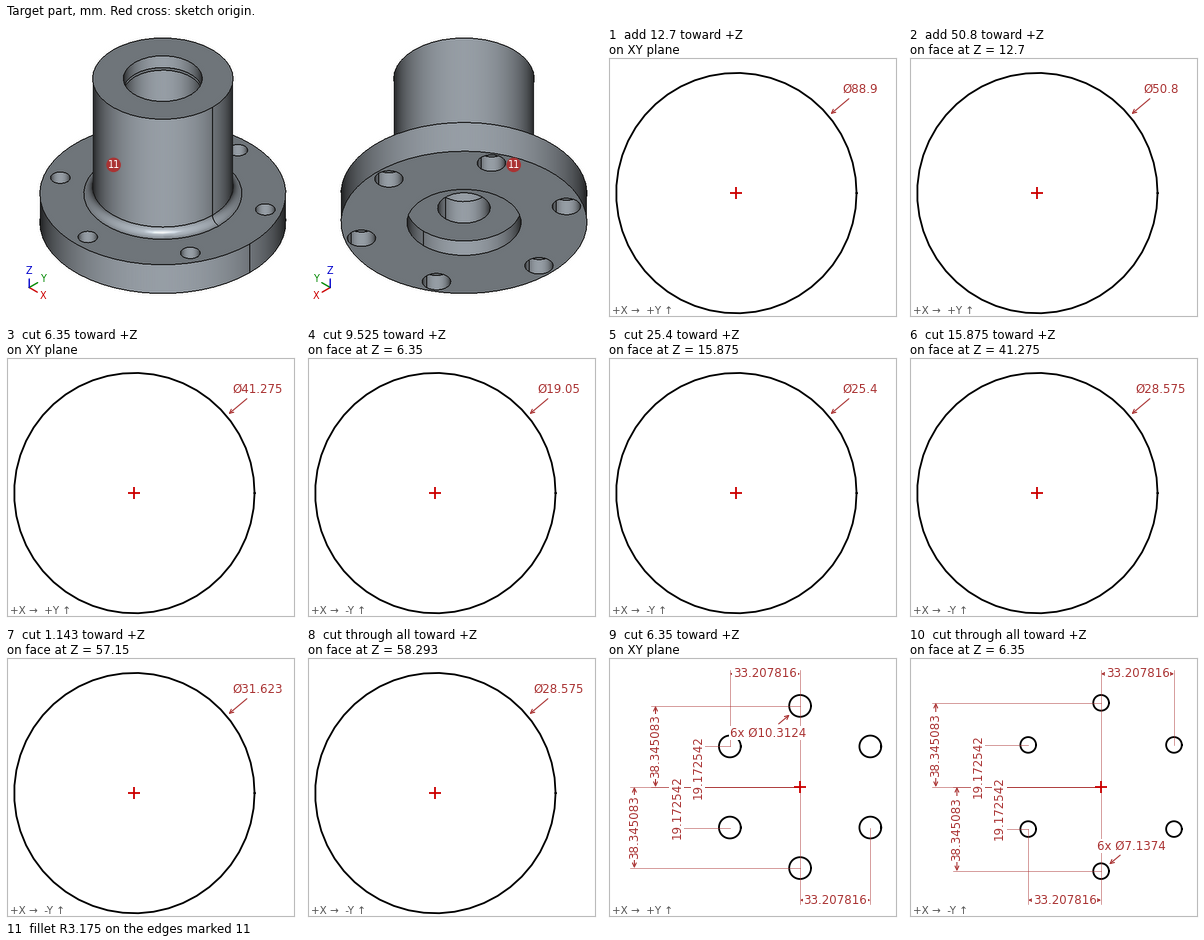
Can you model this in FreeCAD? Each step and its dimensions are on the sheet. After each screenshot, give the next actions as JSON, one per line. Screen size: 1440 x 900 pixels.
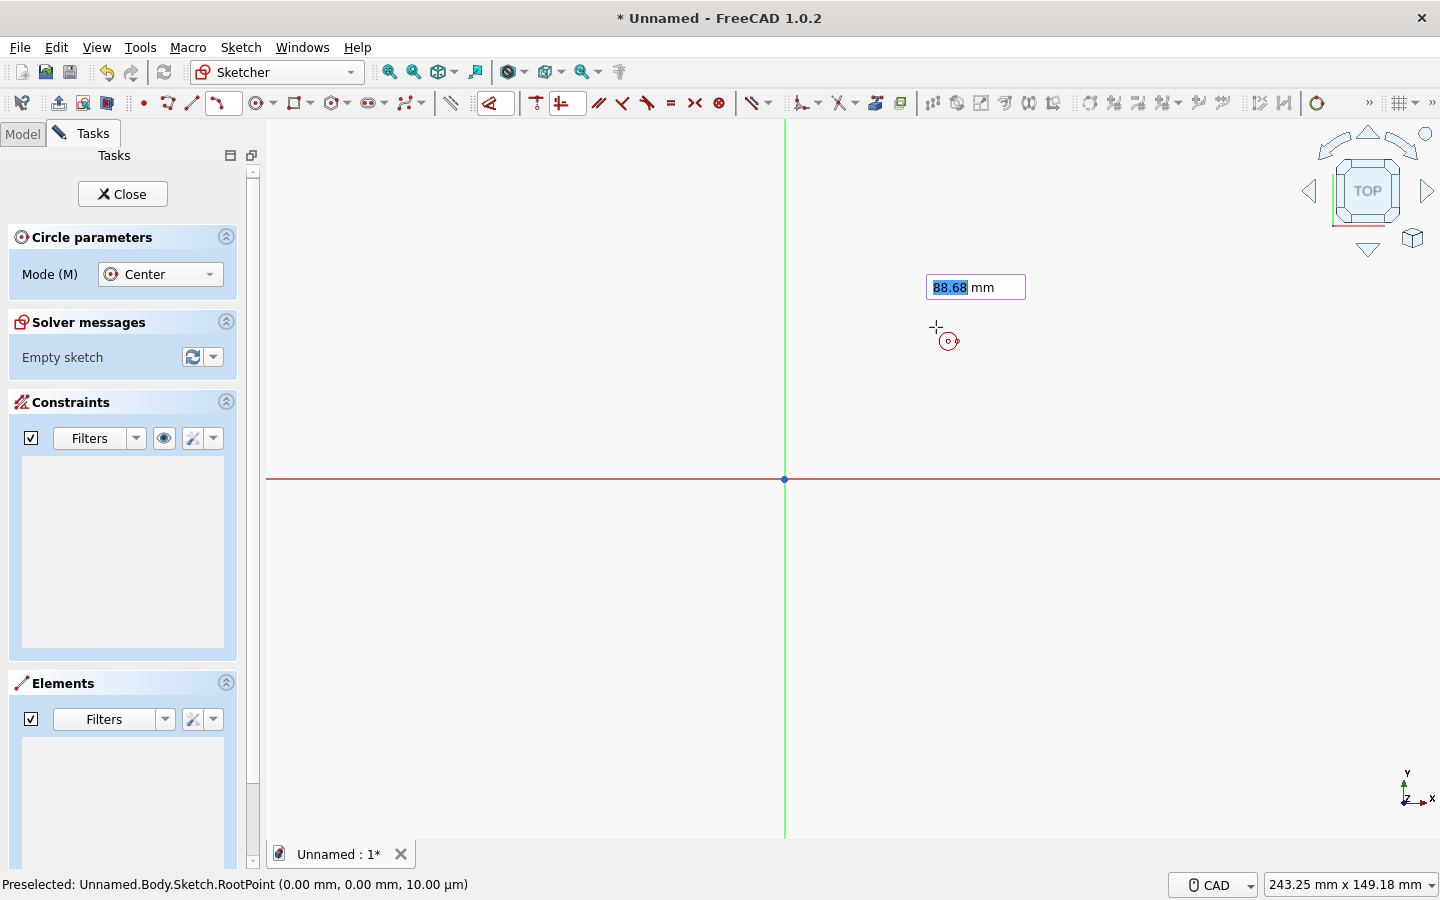
{"action": "type", "text": "88.9"}
{"action": "key", "text": "Return"}
{"action": "key", "text": "Escape"}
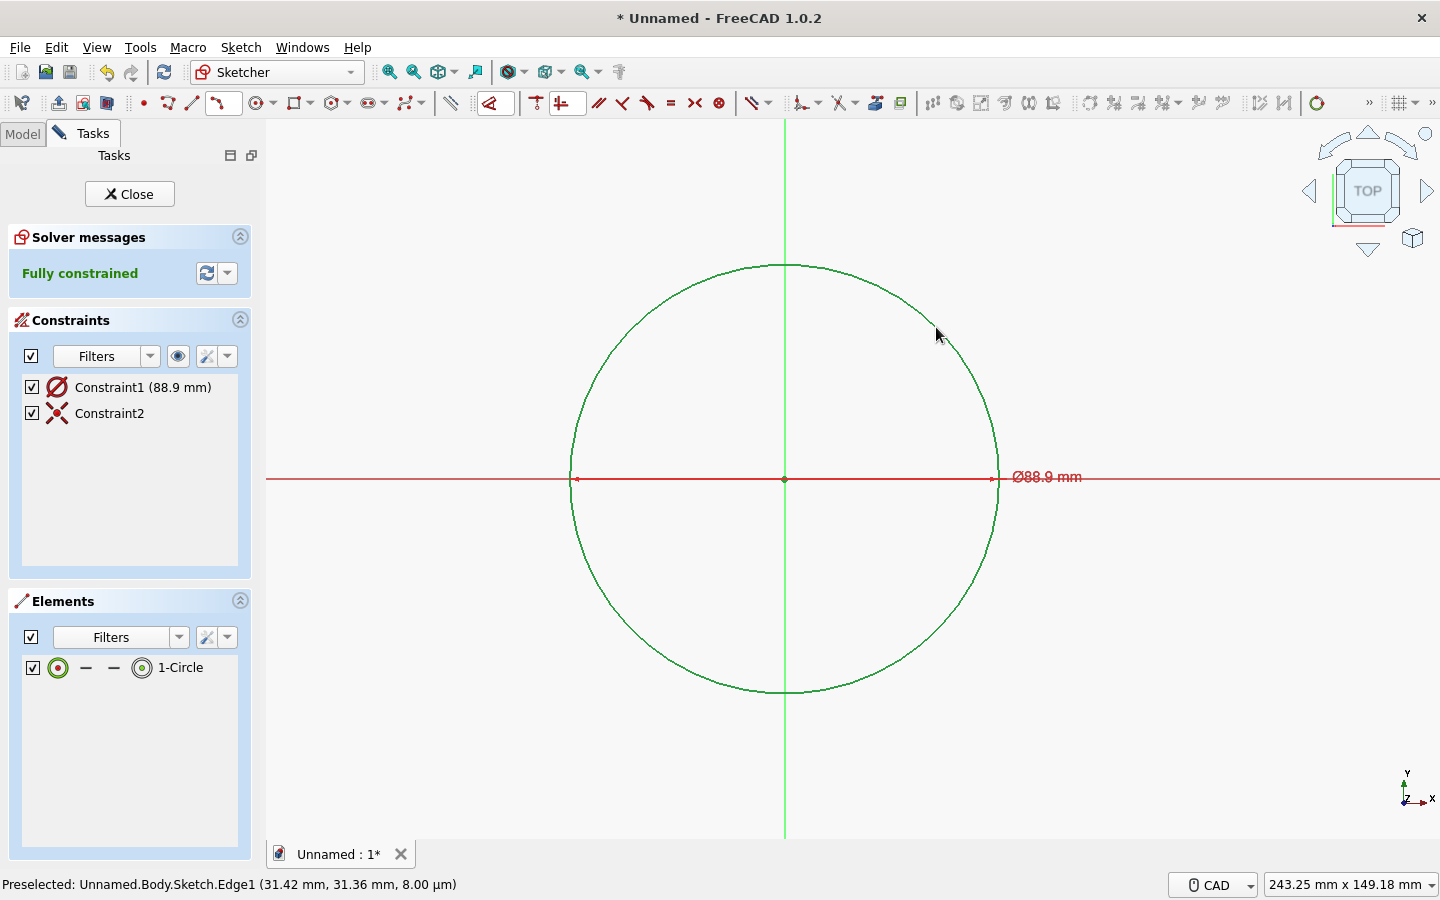
{"action": "left_click", "coordinate": [130, 194]}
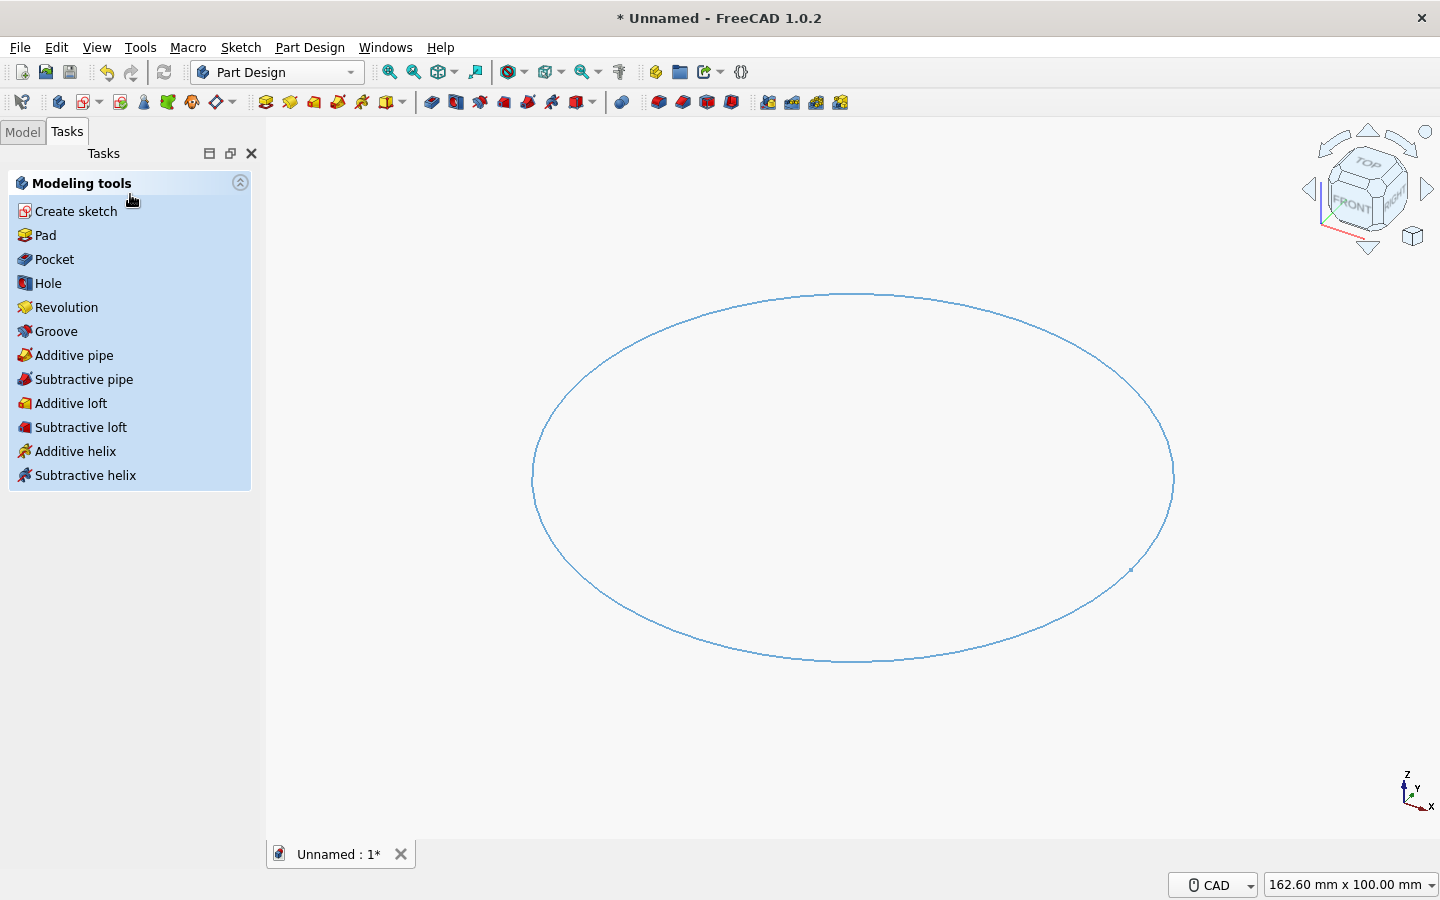
{"action": "left_click", "coordinate": [266, 102]}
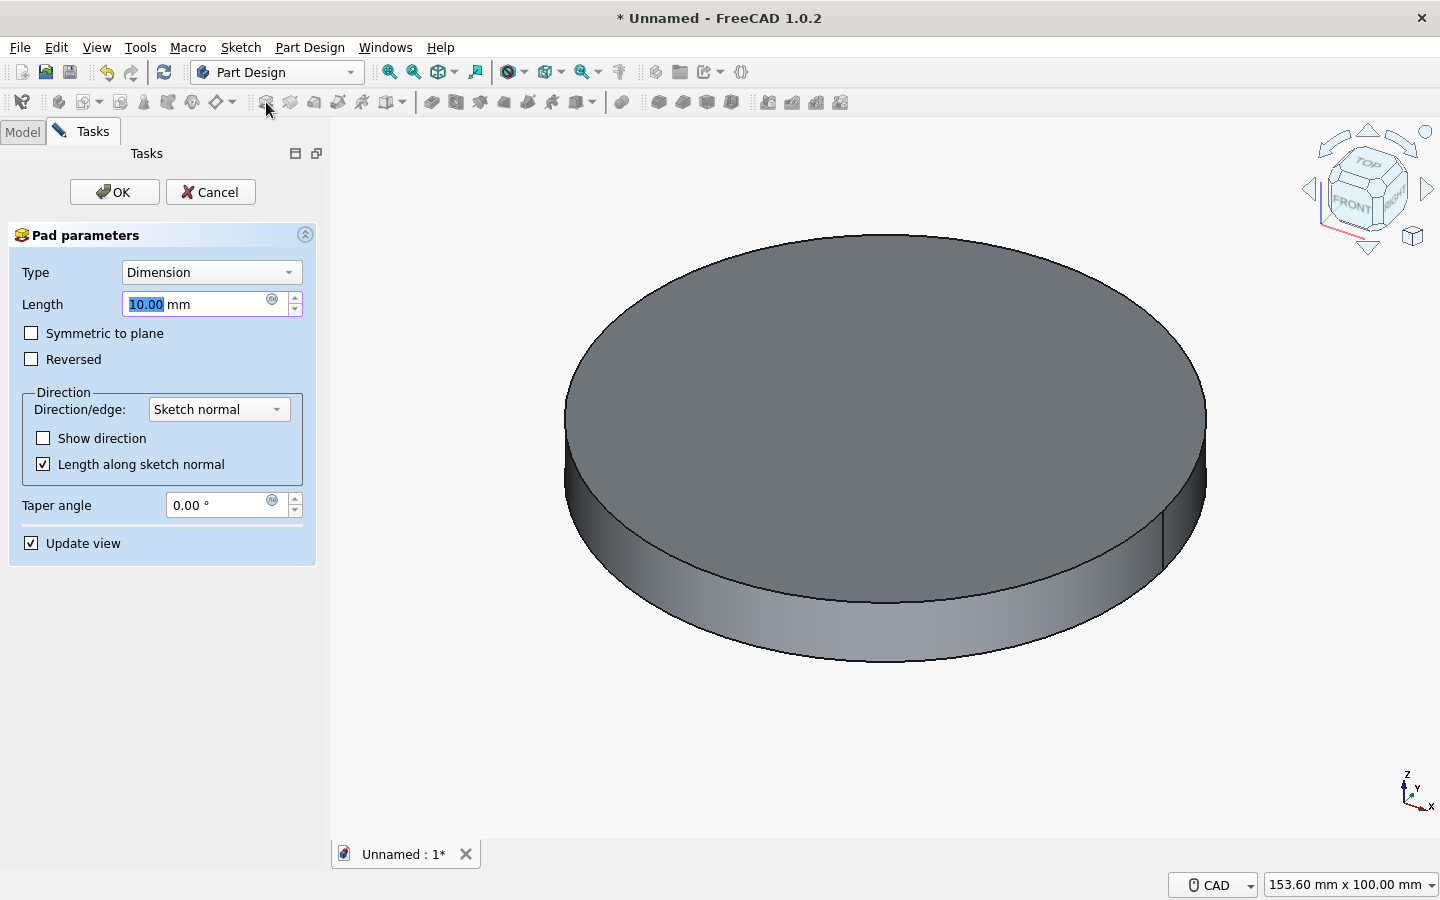
{"action": "type", "text": "12.7"}
{"action": "key", "text": "Tab"}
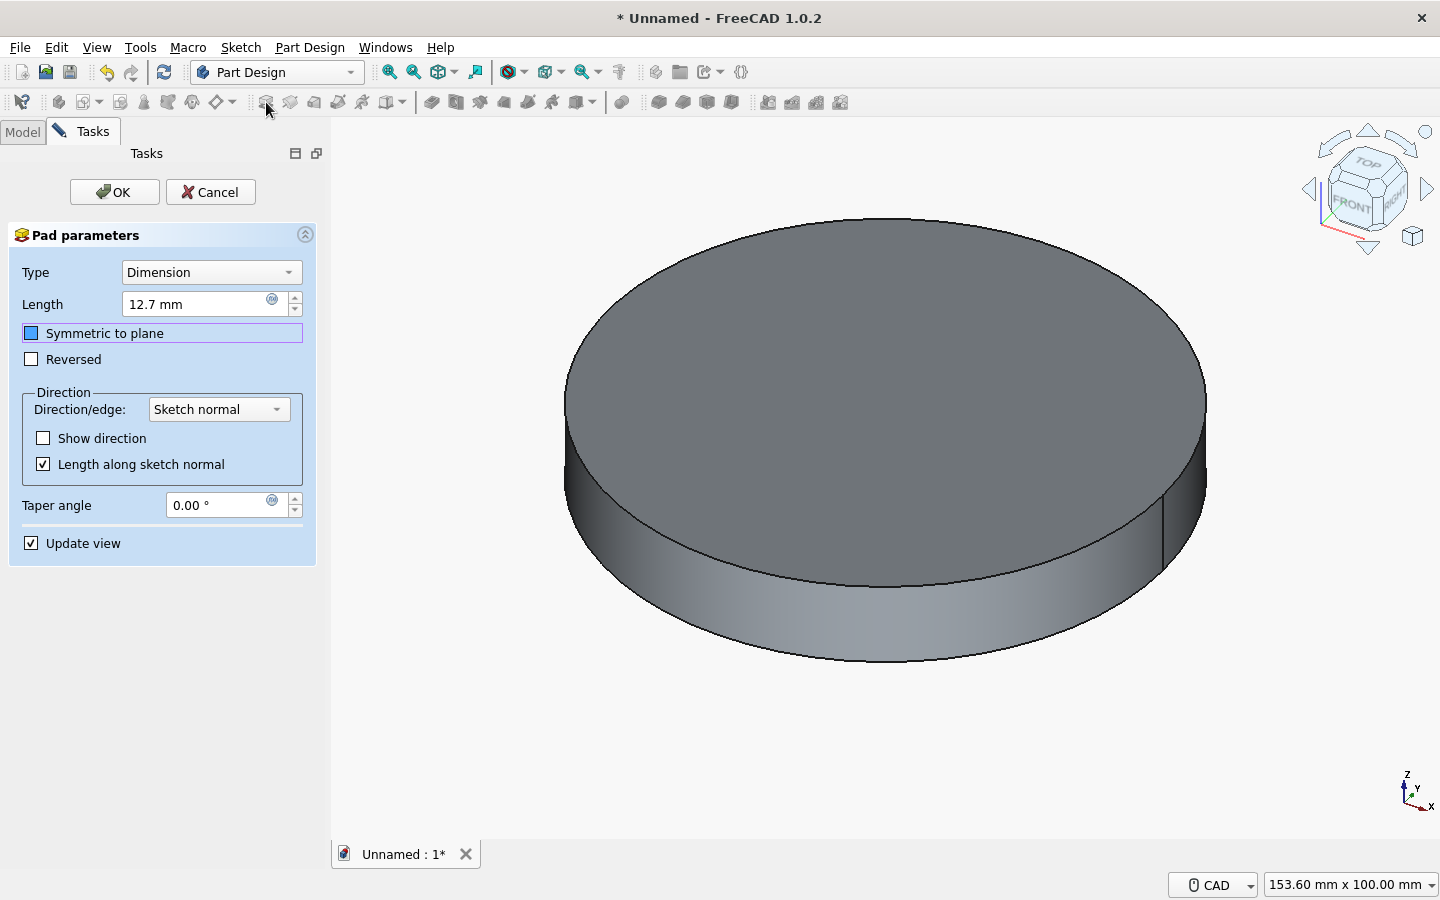
{"action": "left_click", "coordinate": [115, 192]}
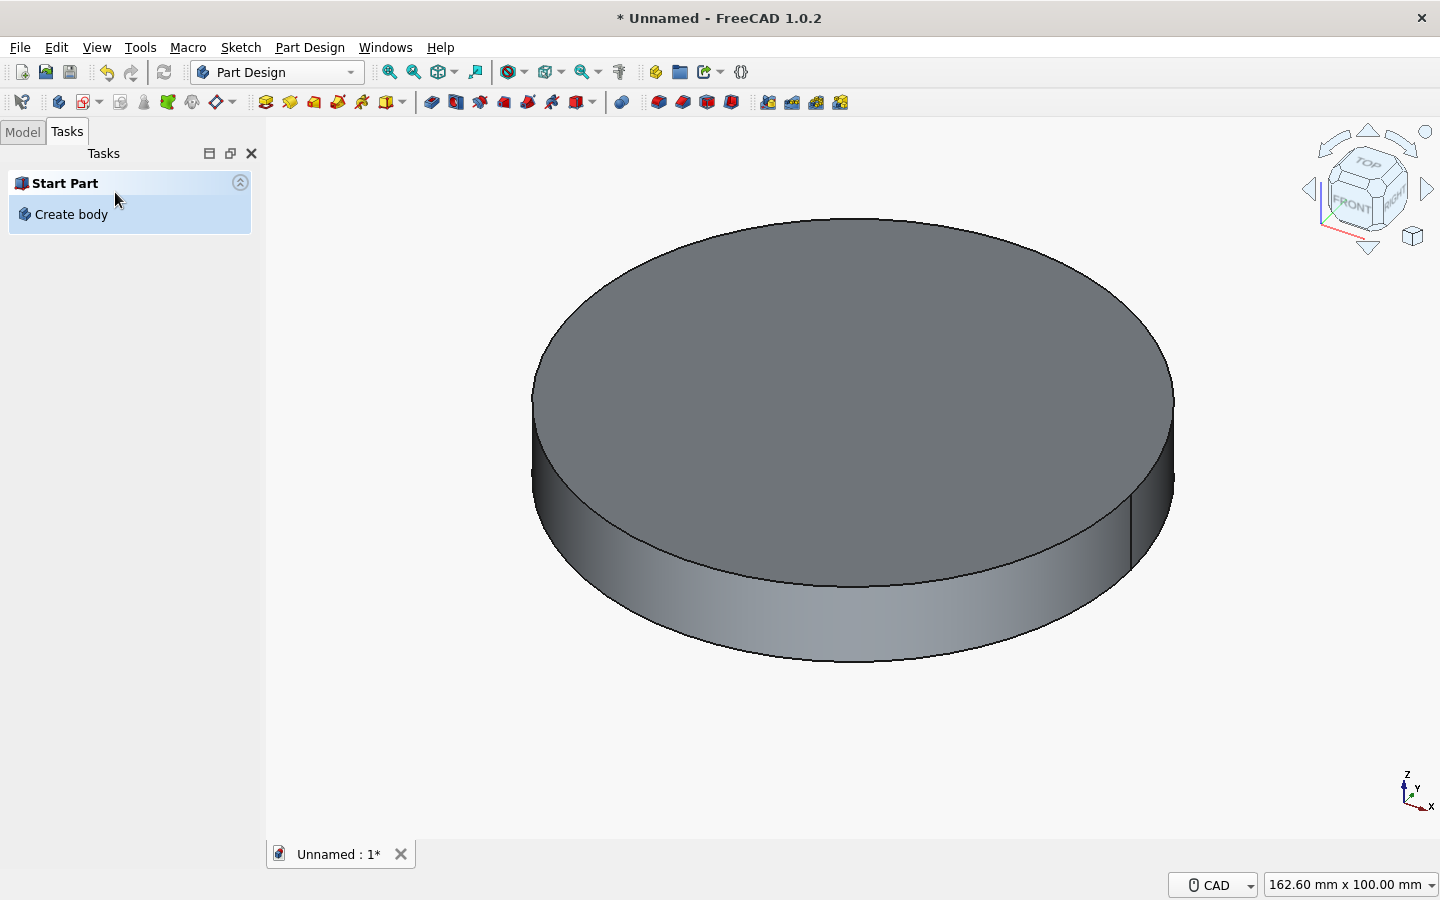
{"action": "left_click", "coordinate": [853, 402]}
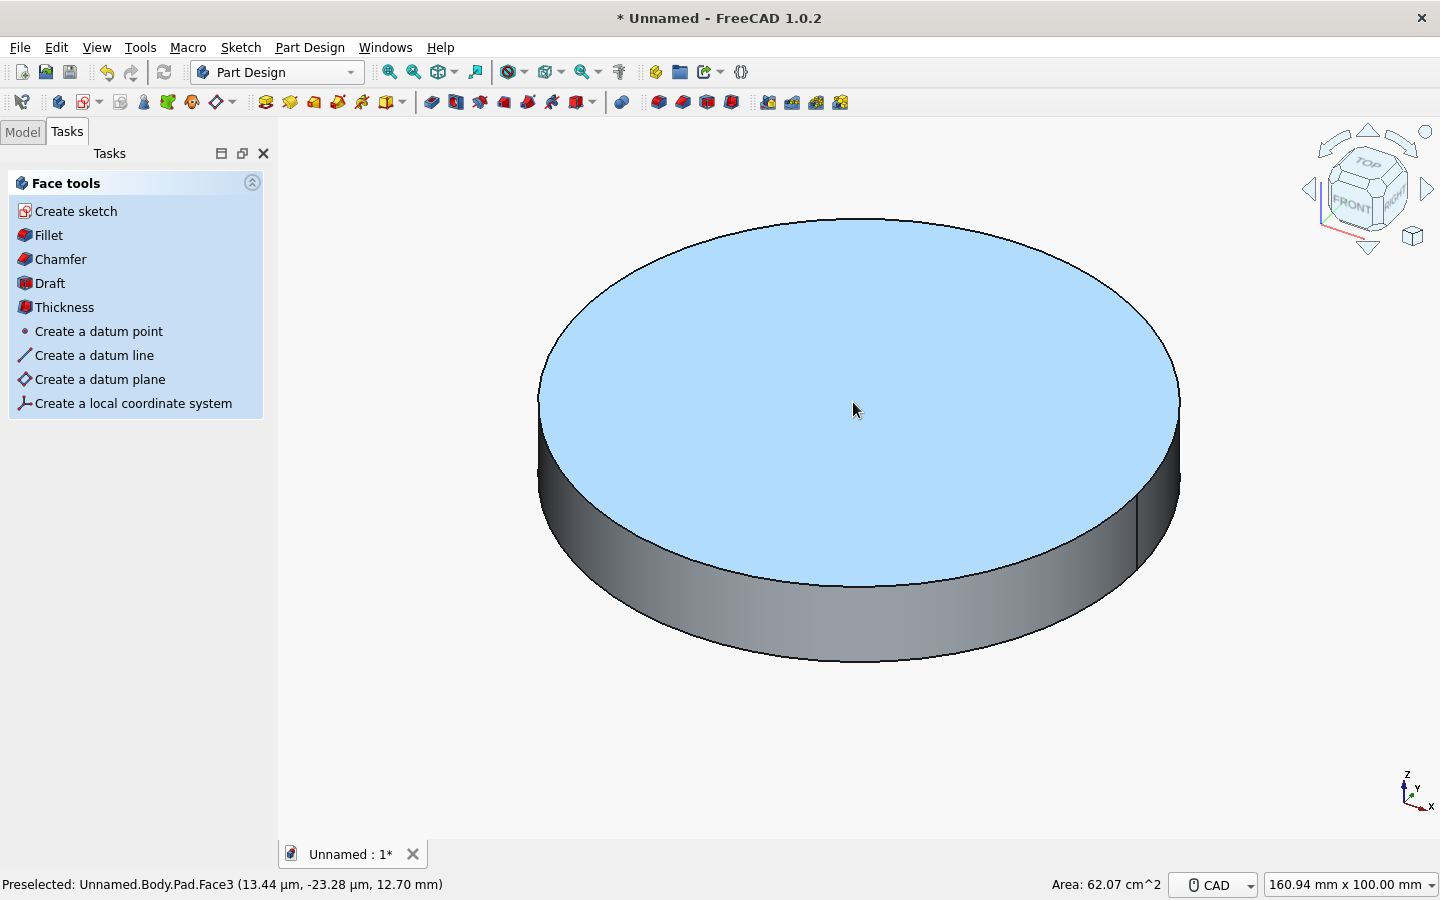
{"action": "left_click", "coordinate": [84, 102]}